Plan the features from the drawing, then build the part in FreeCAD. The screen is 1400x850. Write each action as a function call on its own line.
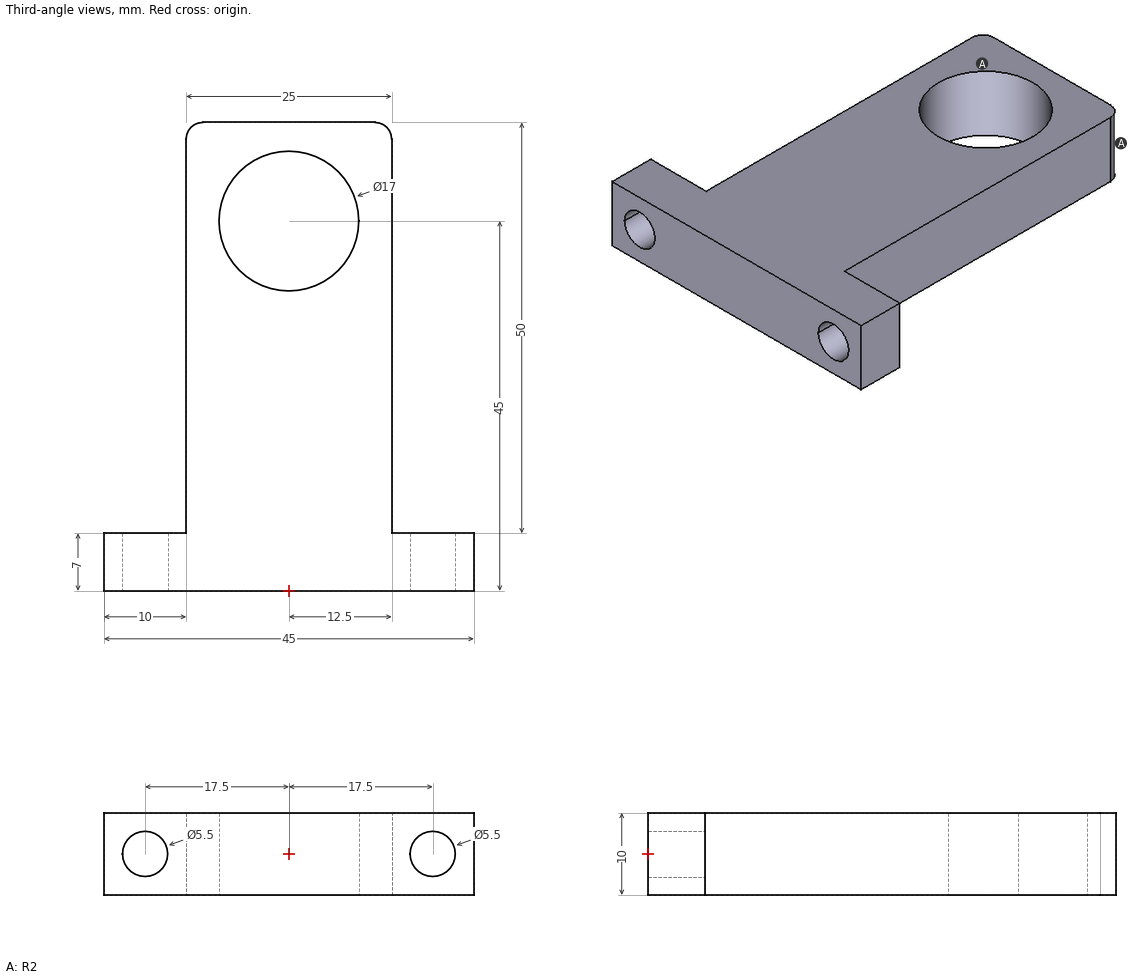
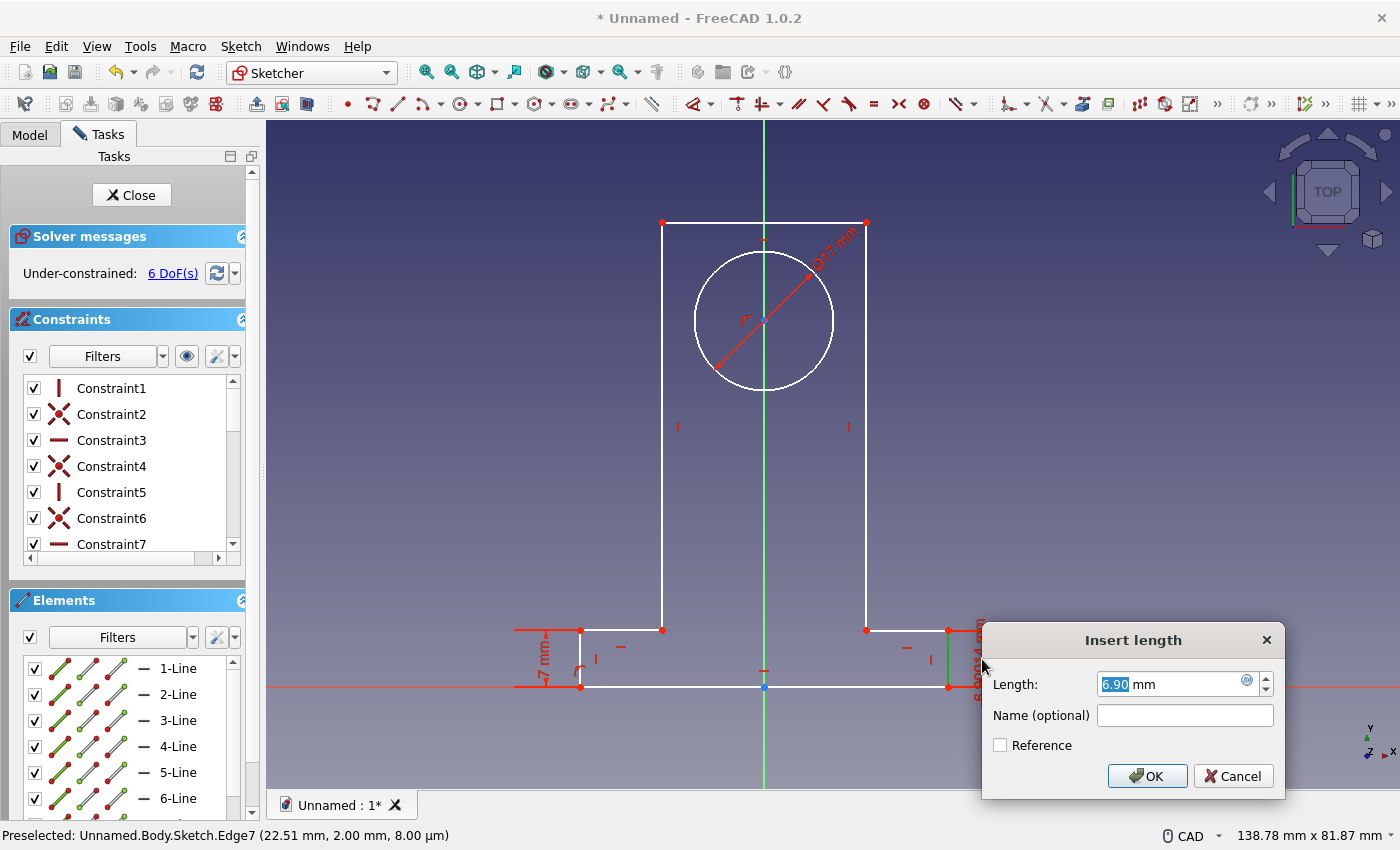
text(7)
key(Return)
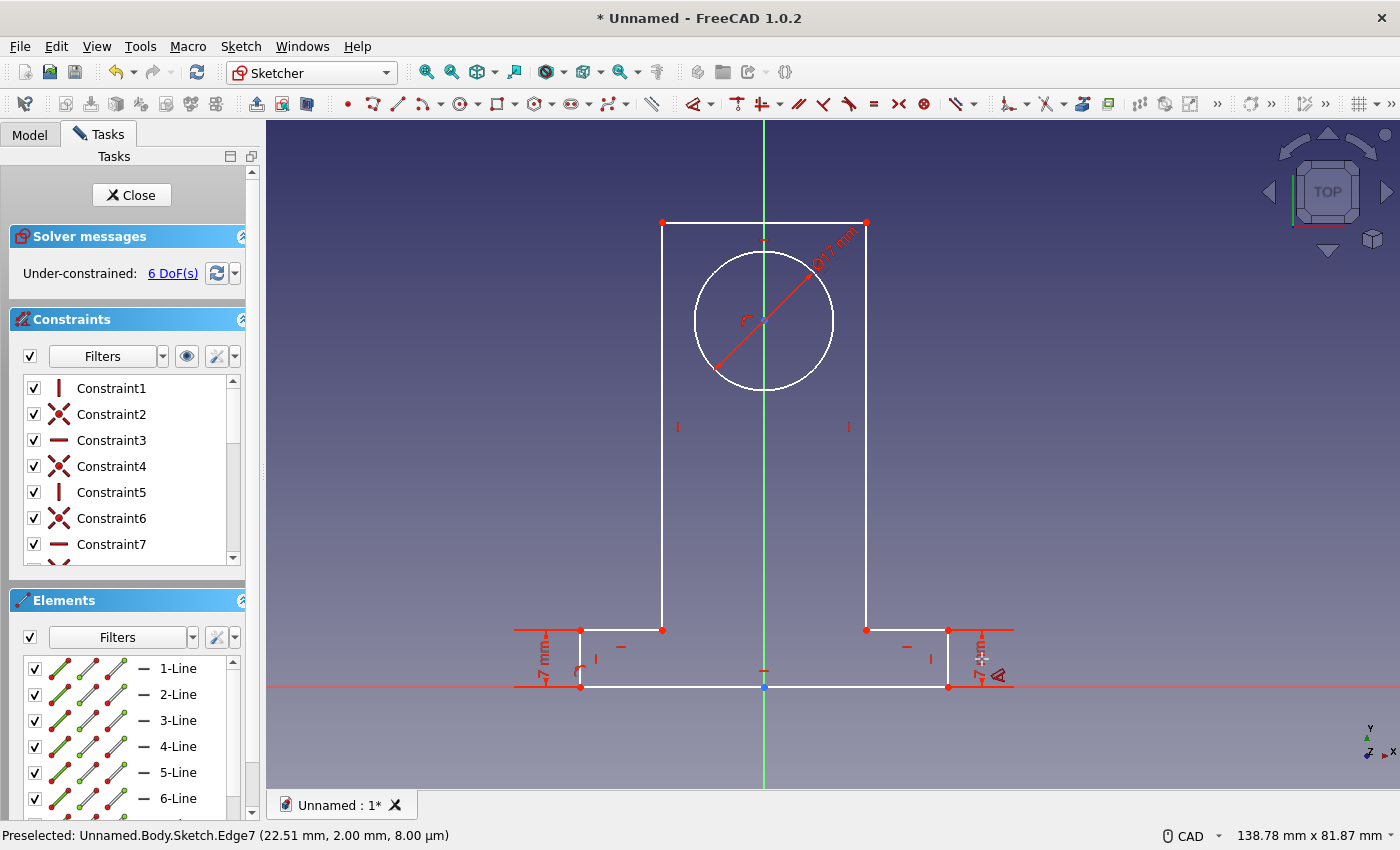
click(866, 508)
click(900, 427)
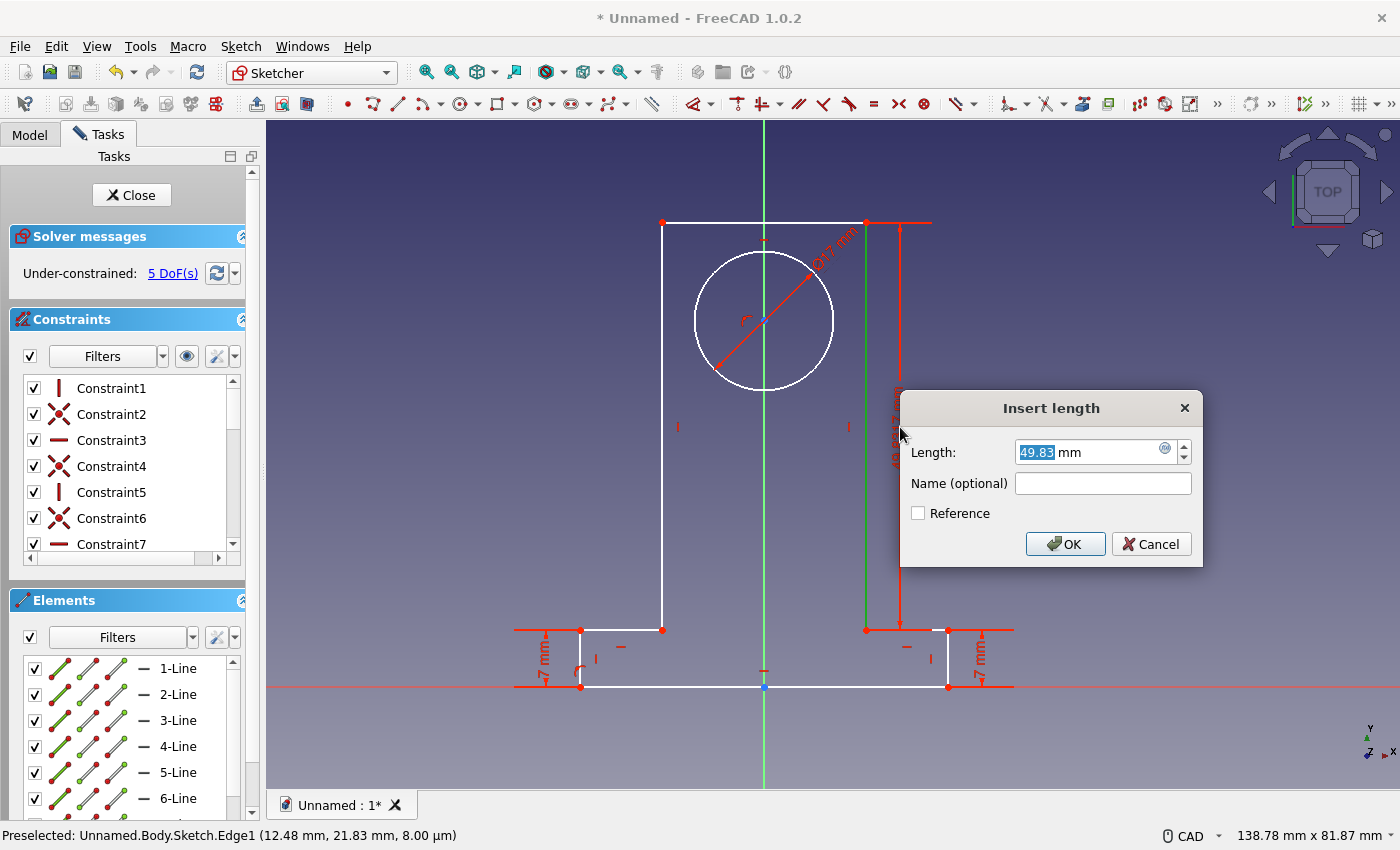
text(50)
key(Return)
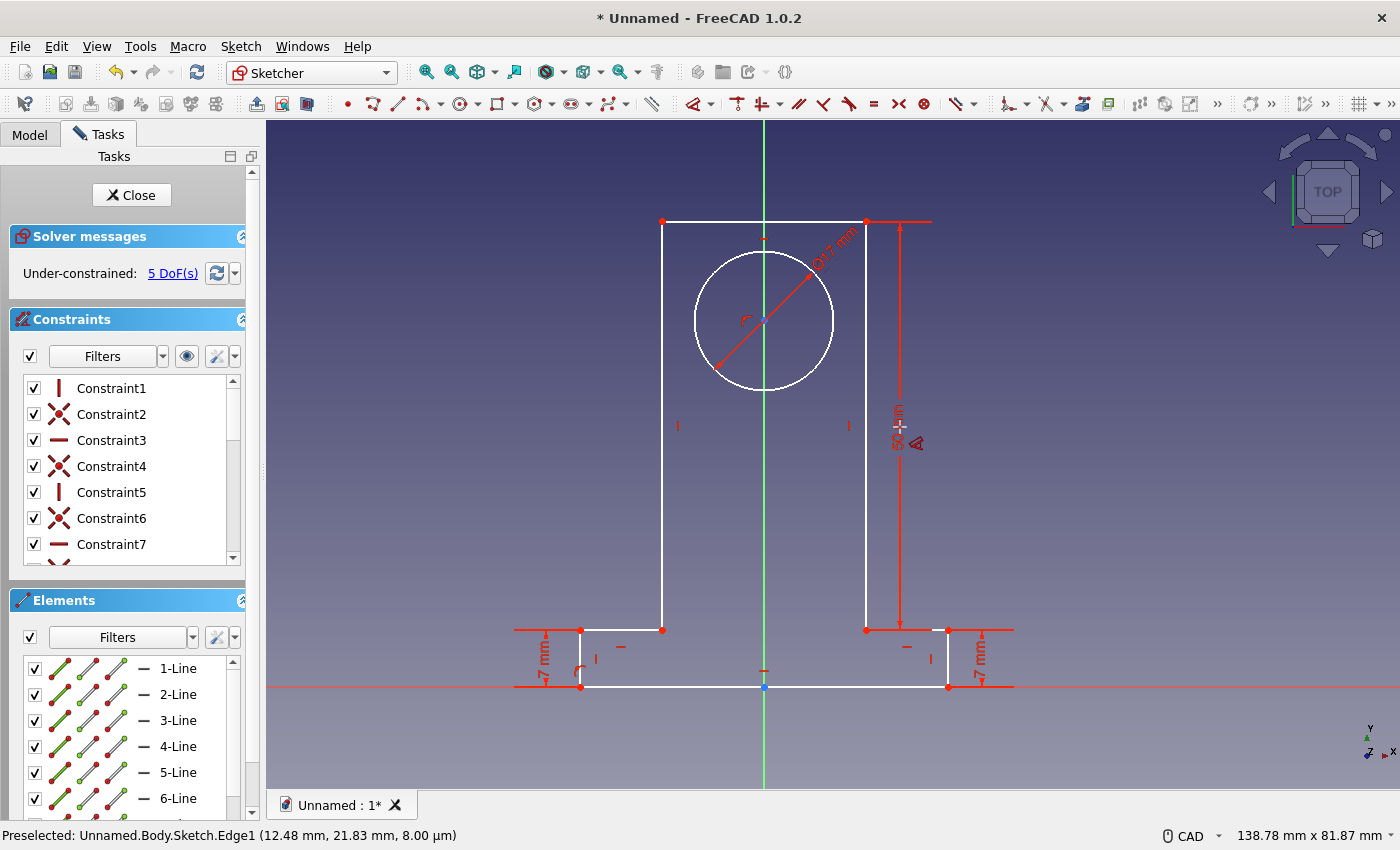
click(805, 222)
click(717, 188)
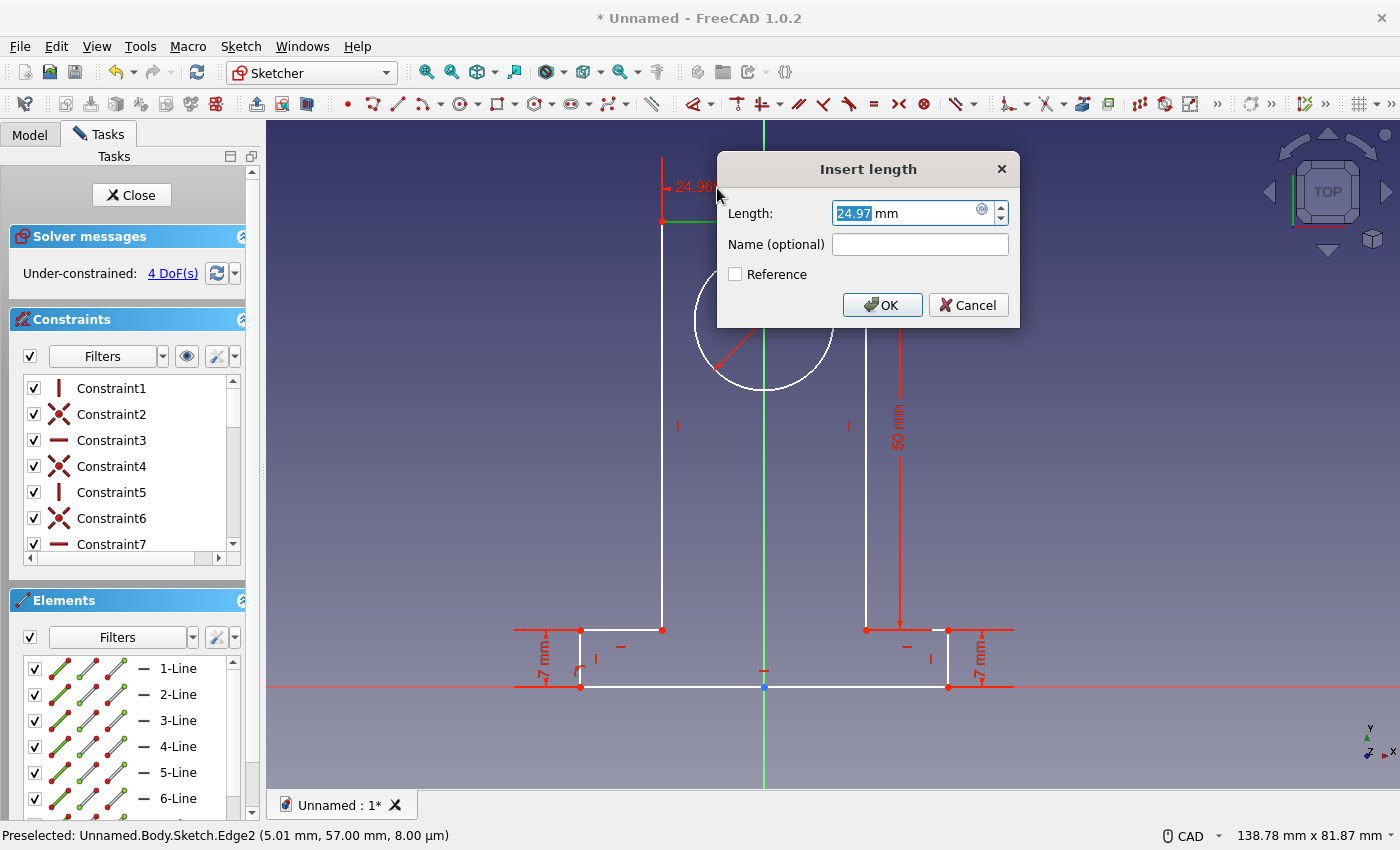
text(25)
key(Return)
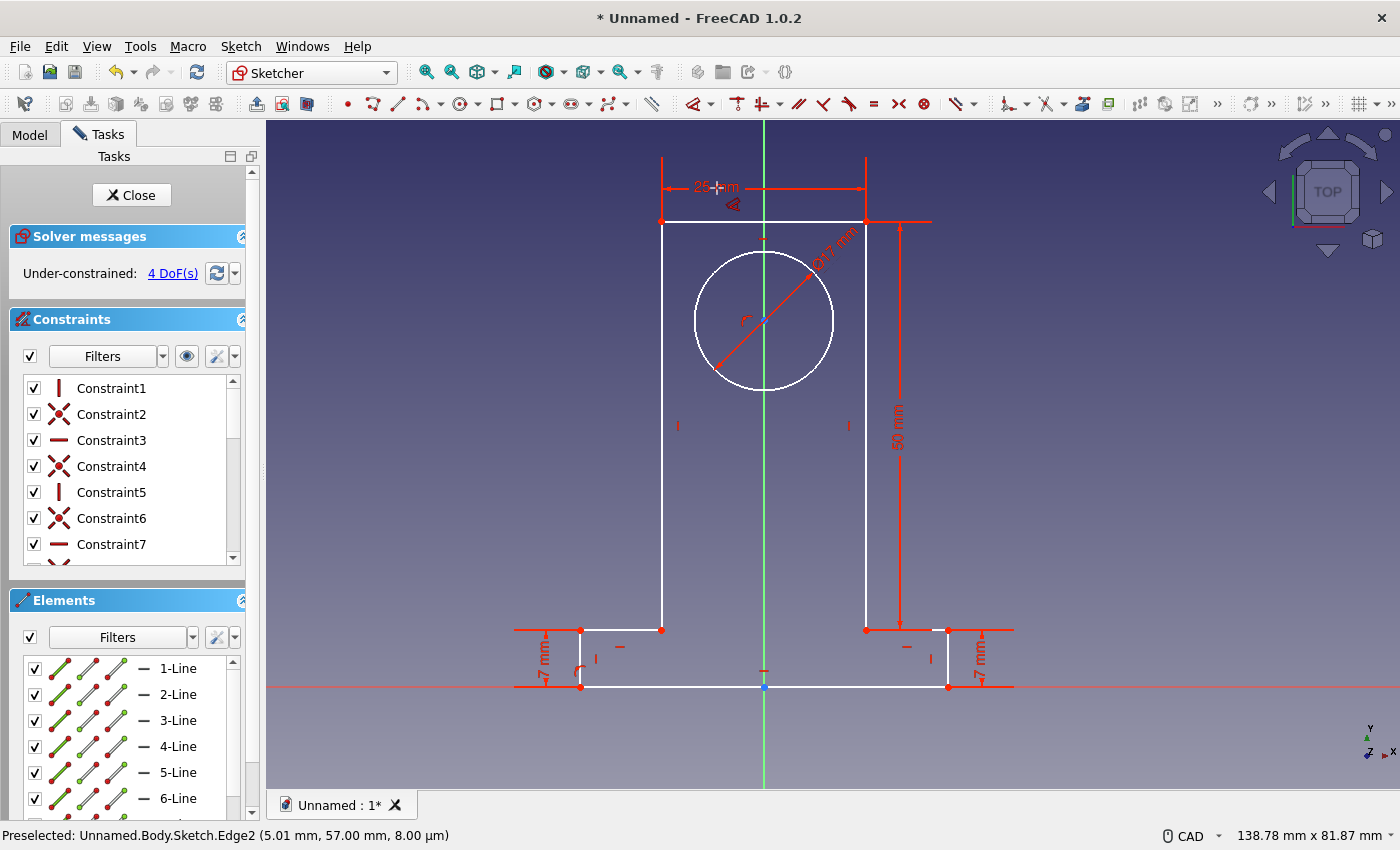
click(637, 630)
click(621, 664)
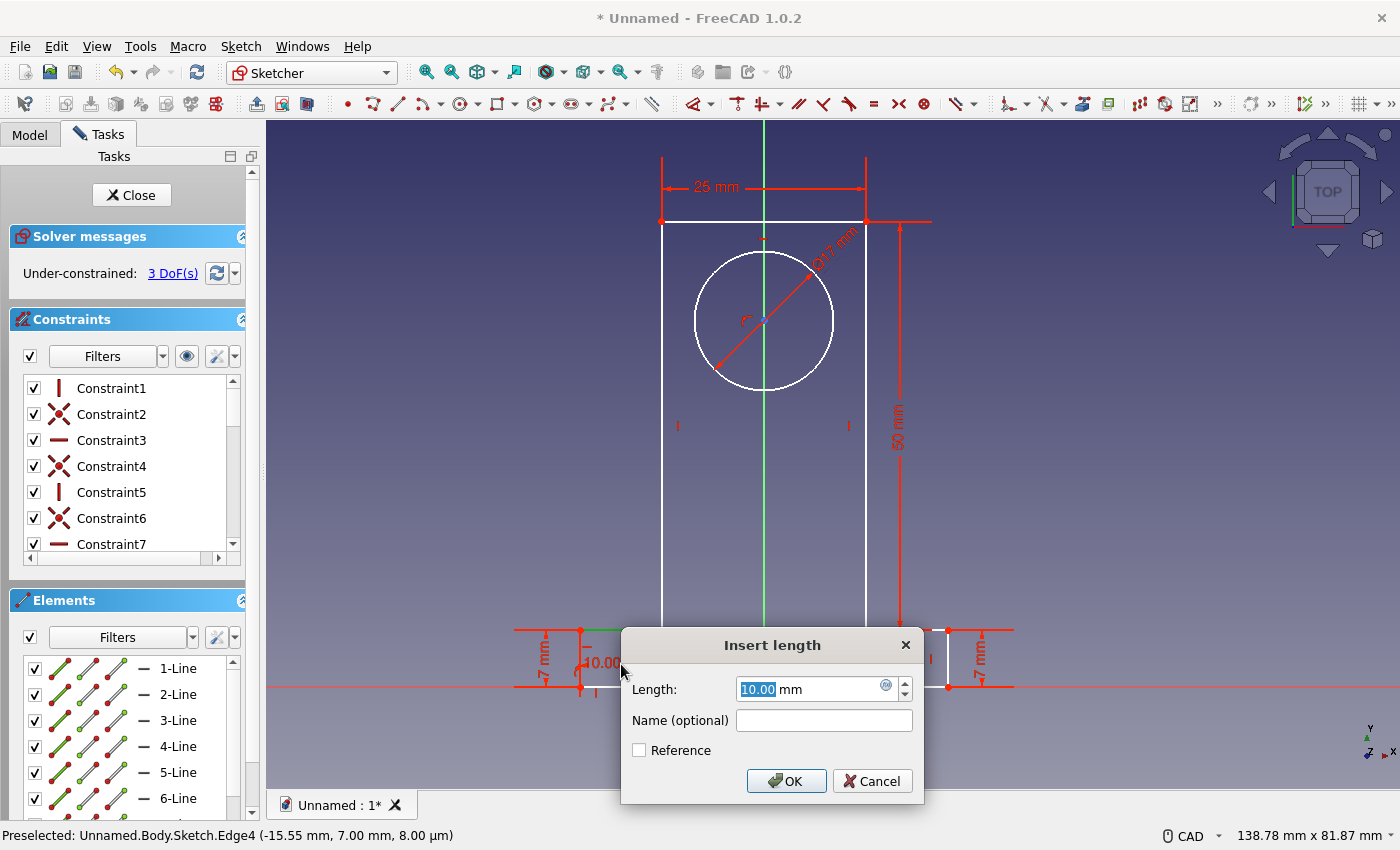
text(10)
key(Return)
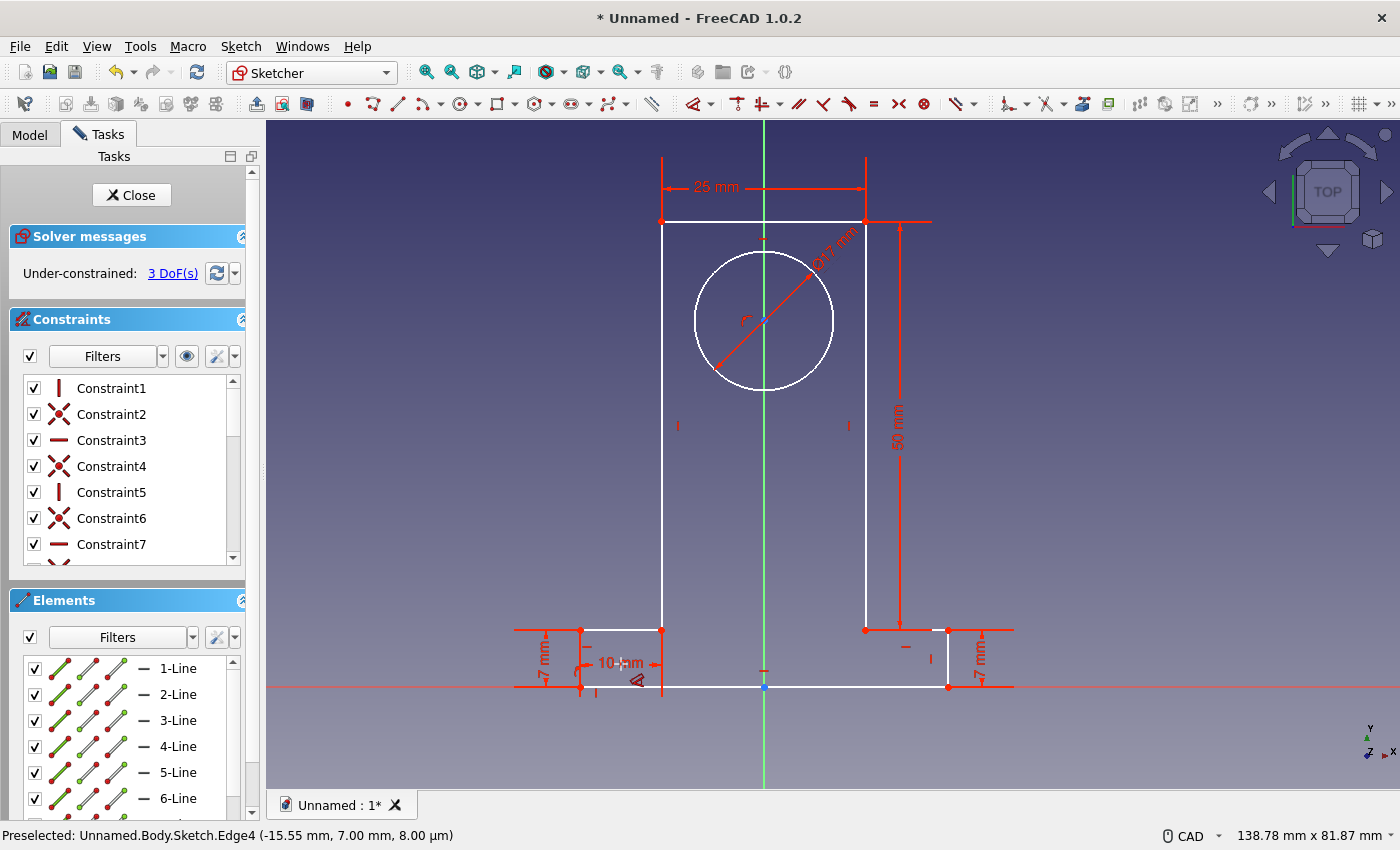
click(690, 687)
click(679, 721)